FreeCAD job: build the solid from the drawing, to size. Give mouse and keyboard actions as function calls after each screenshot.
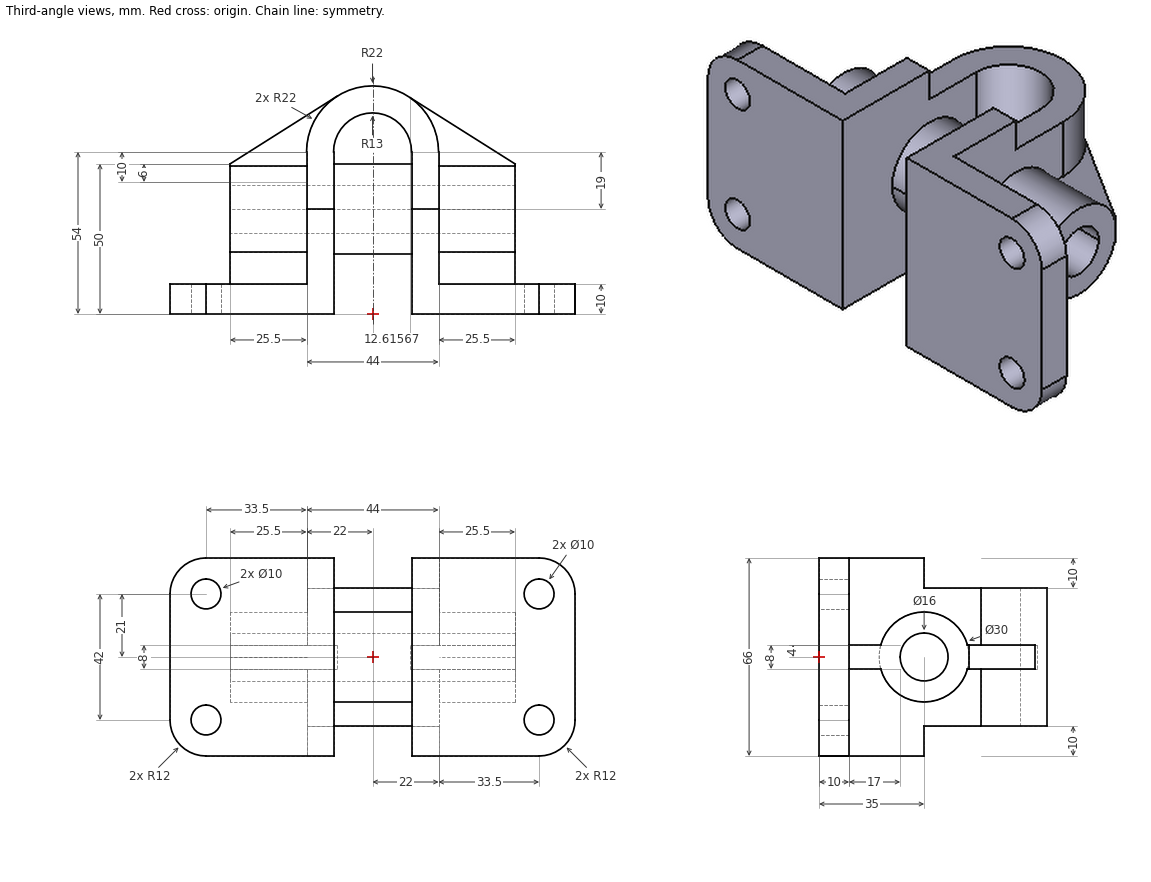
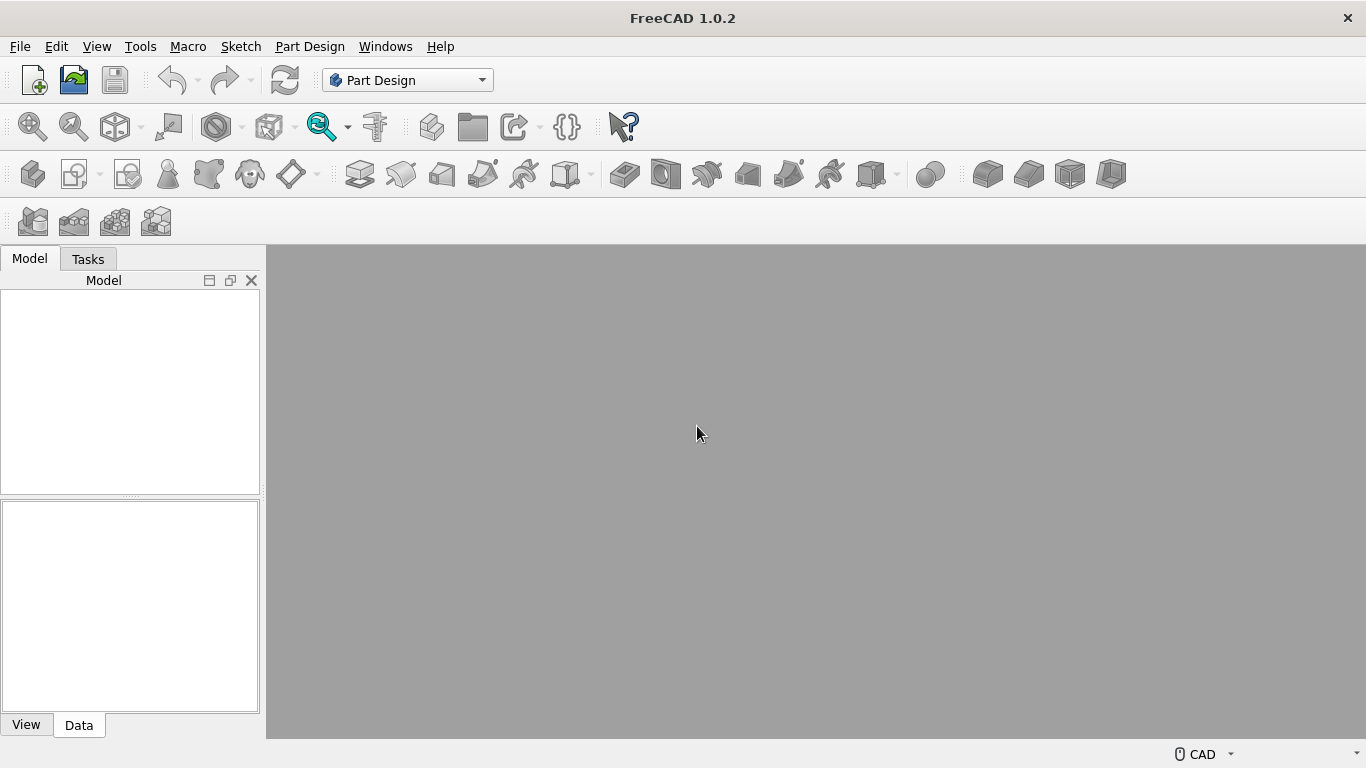
click(33, 80)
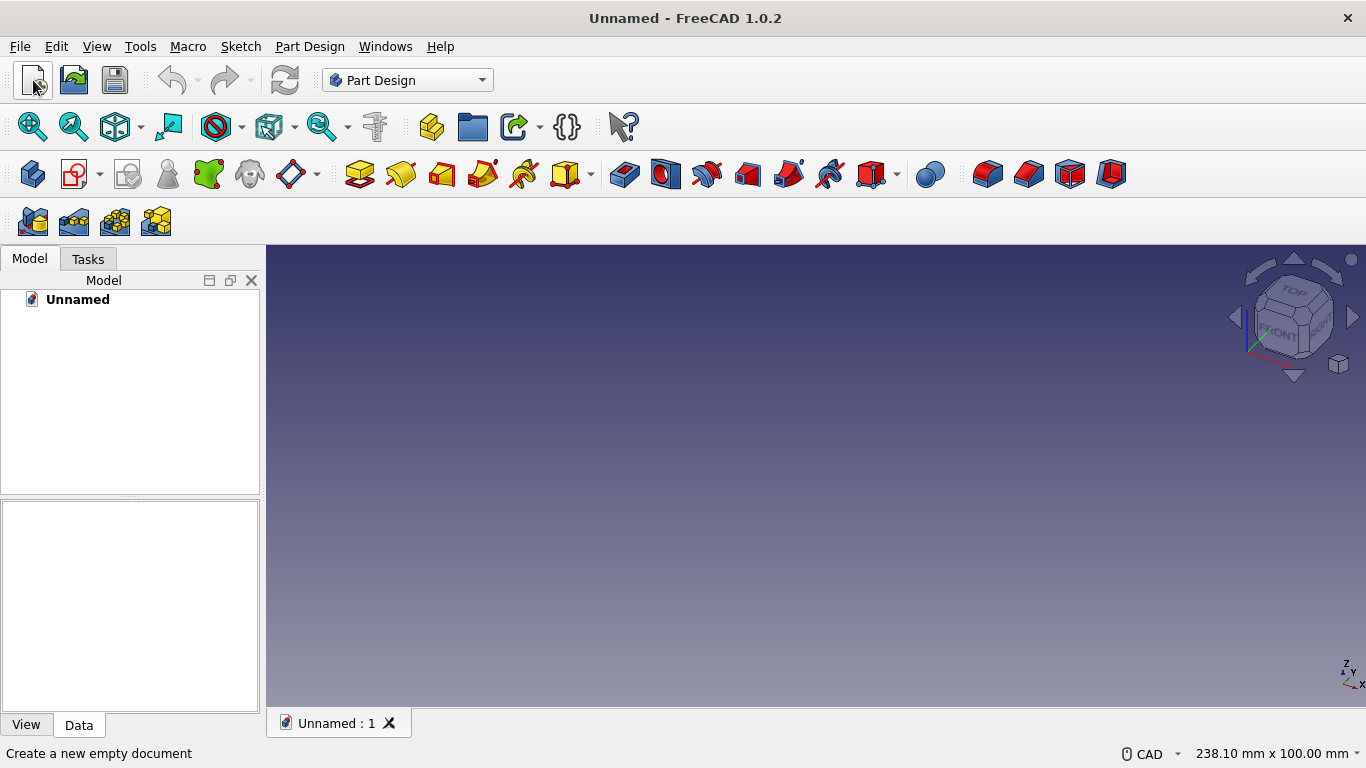
click(74, 174)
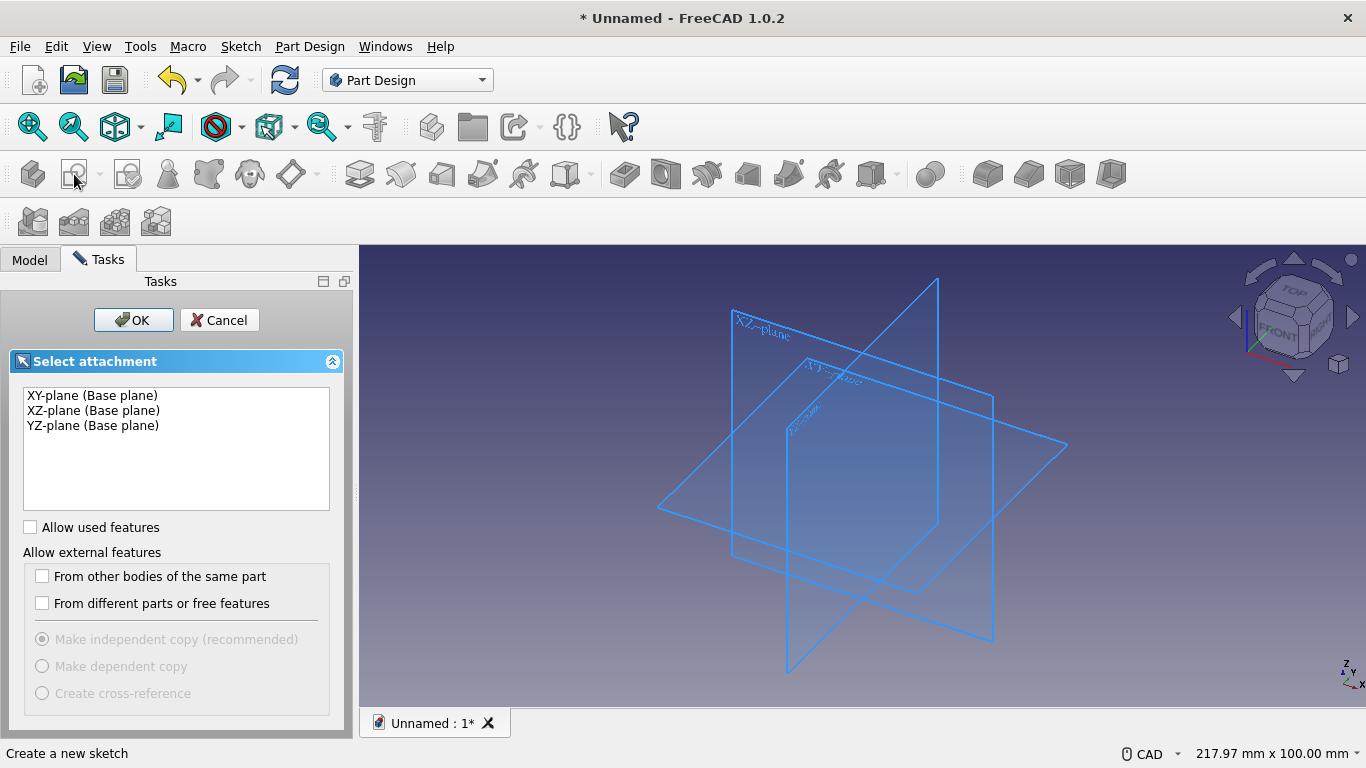
click(84, 410)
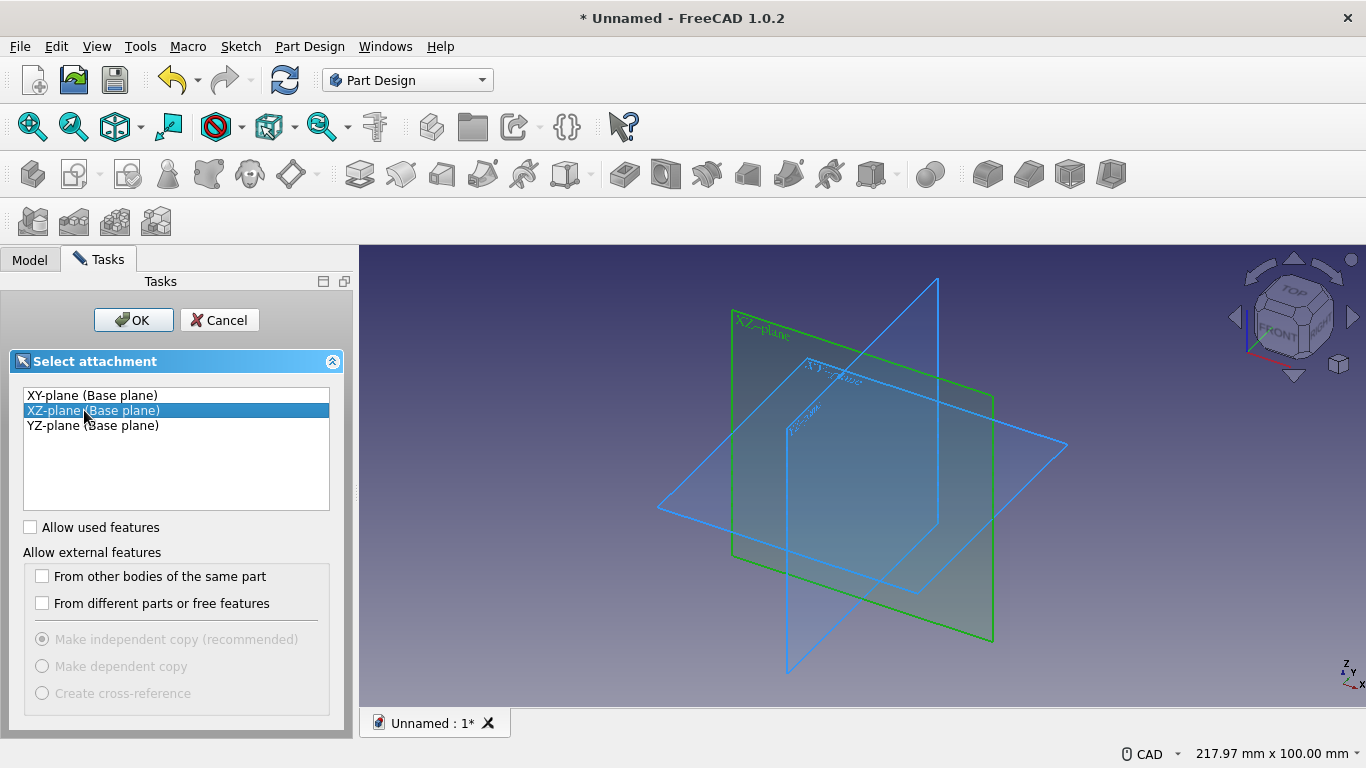
click(134, 320)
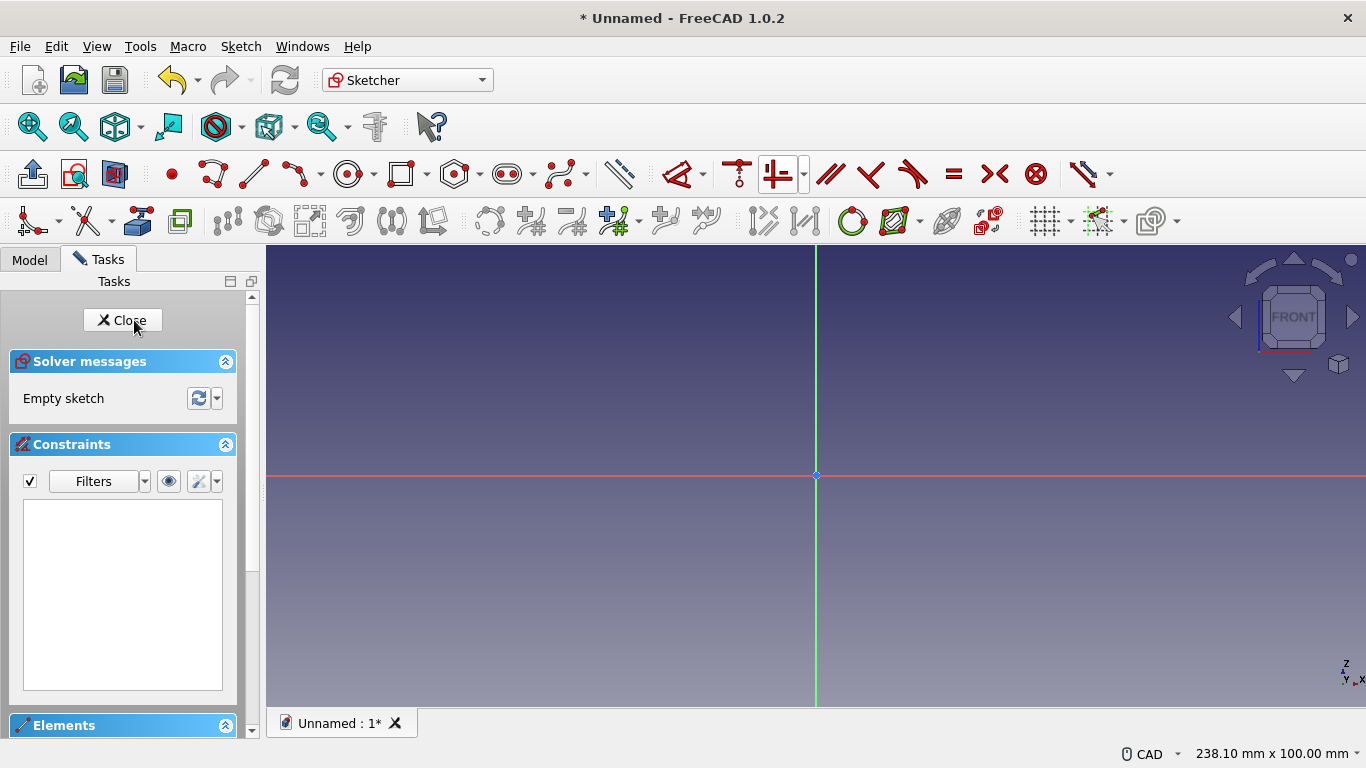
click(254, 174)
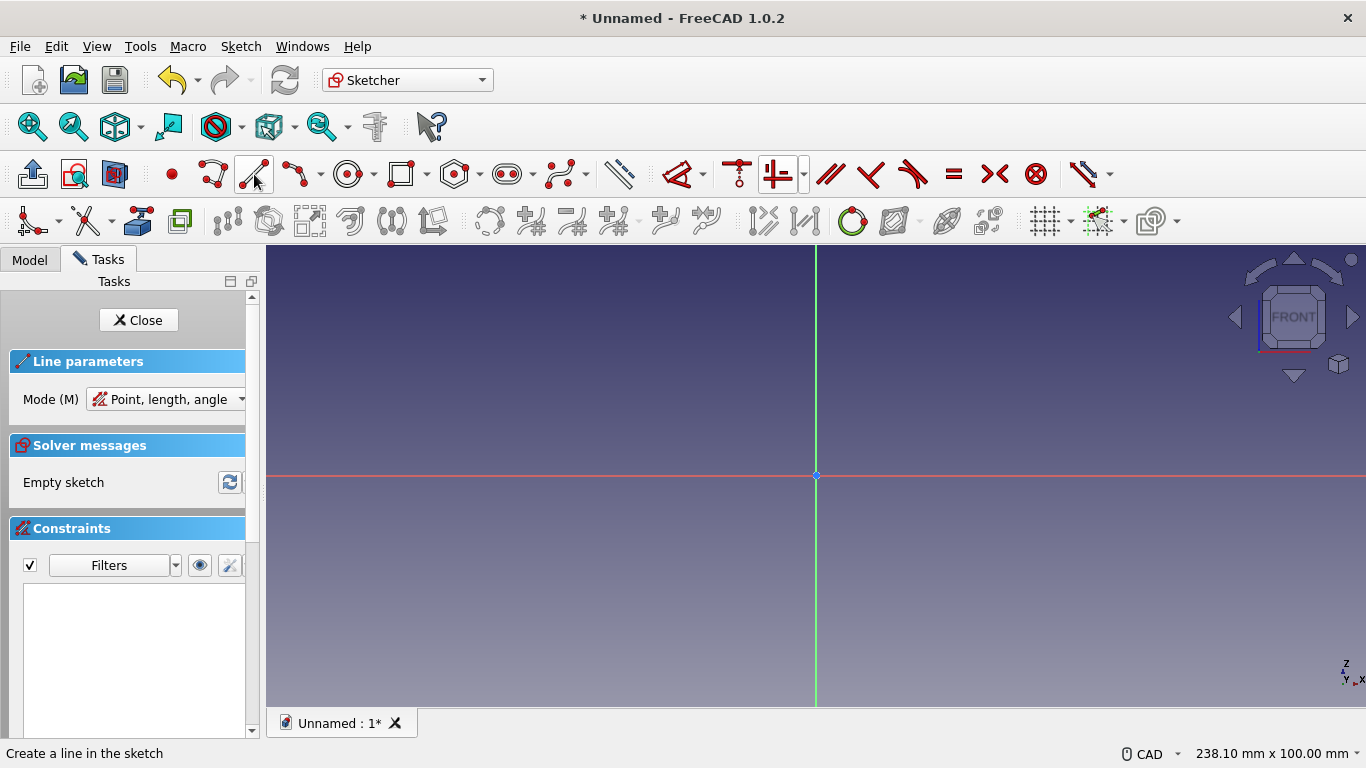
click(504, 573)
click(504, 379)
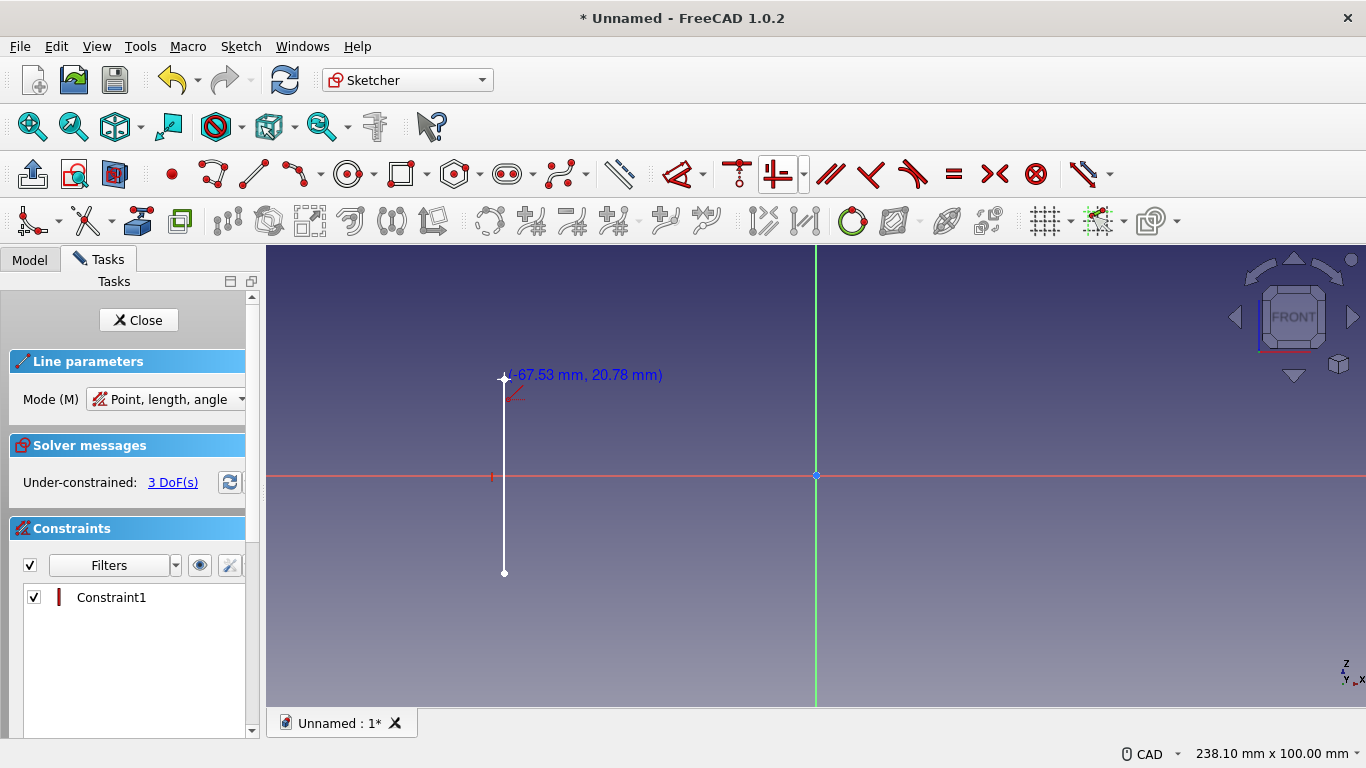
click(213, 174)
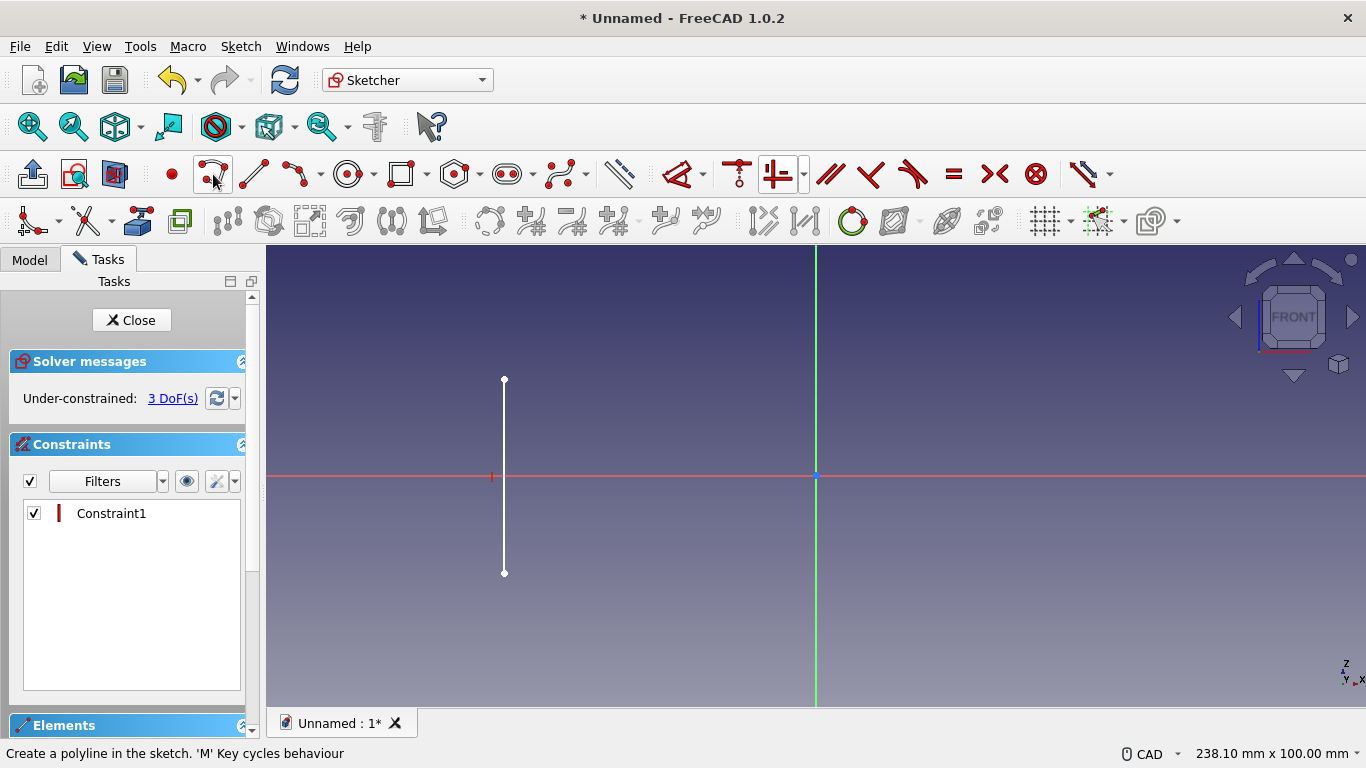
click(560, 324)
click(714, 324)
click(714, 628)
click(560, 628)
right_click(560, 628)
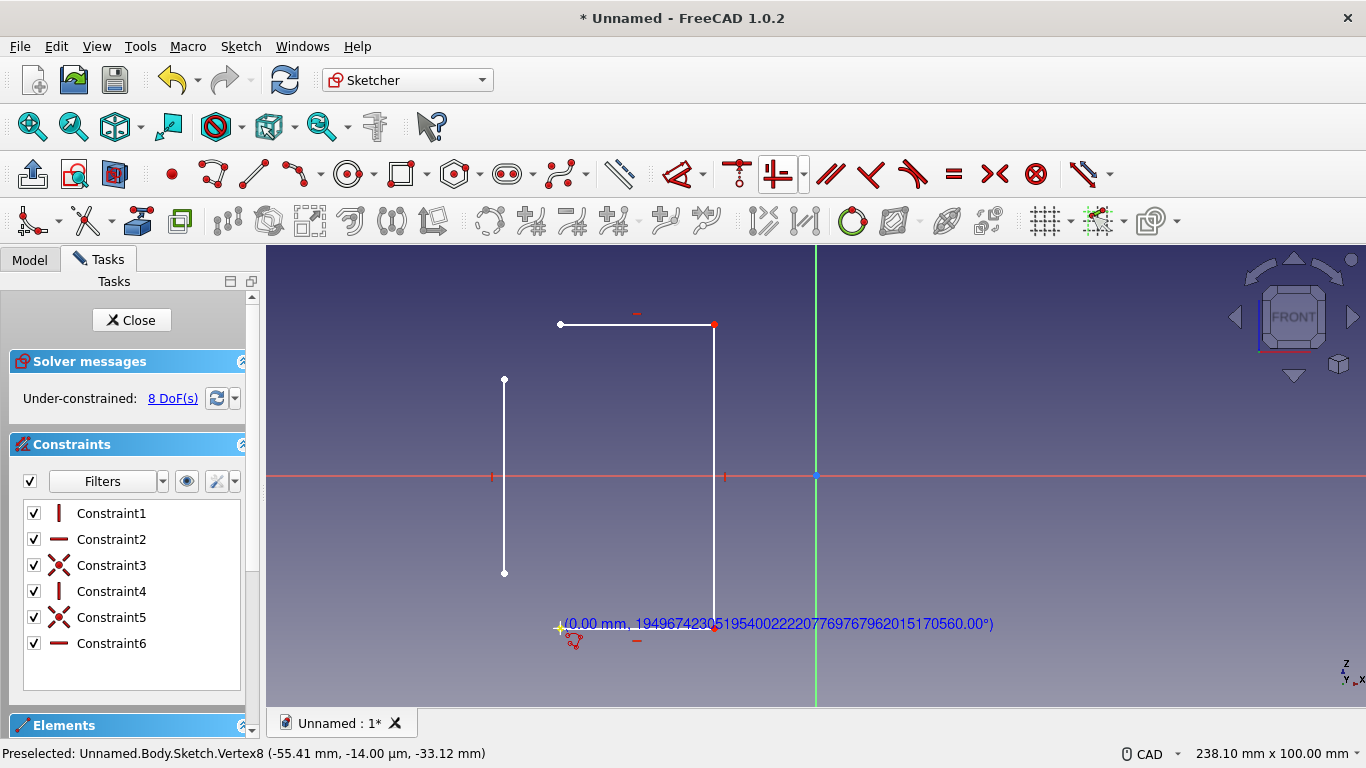
click(294, 174)